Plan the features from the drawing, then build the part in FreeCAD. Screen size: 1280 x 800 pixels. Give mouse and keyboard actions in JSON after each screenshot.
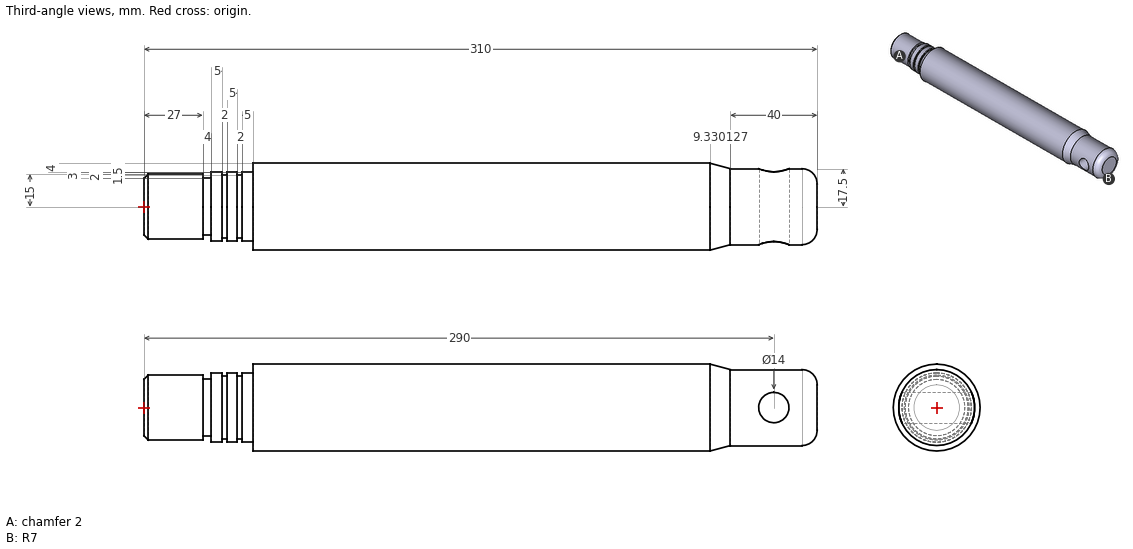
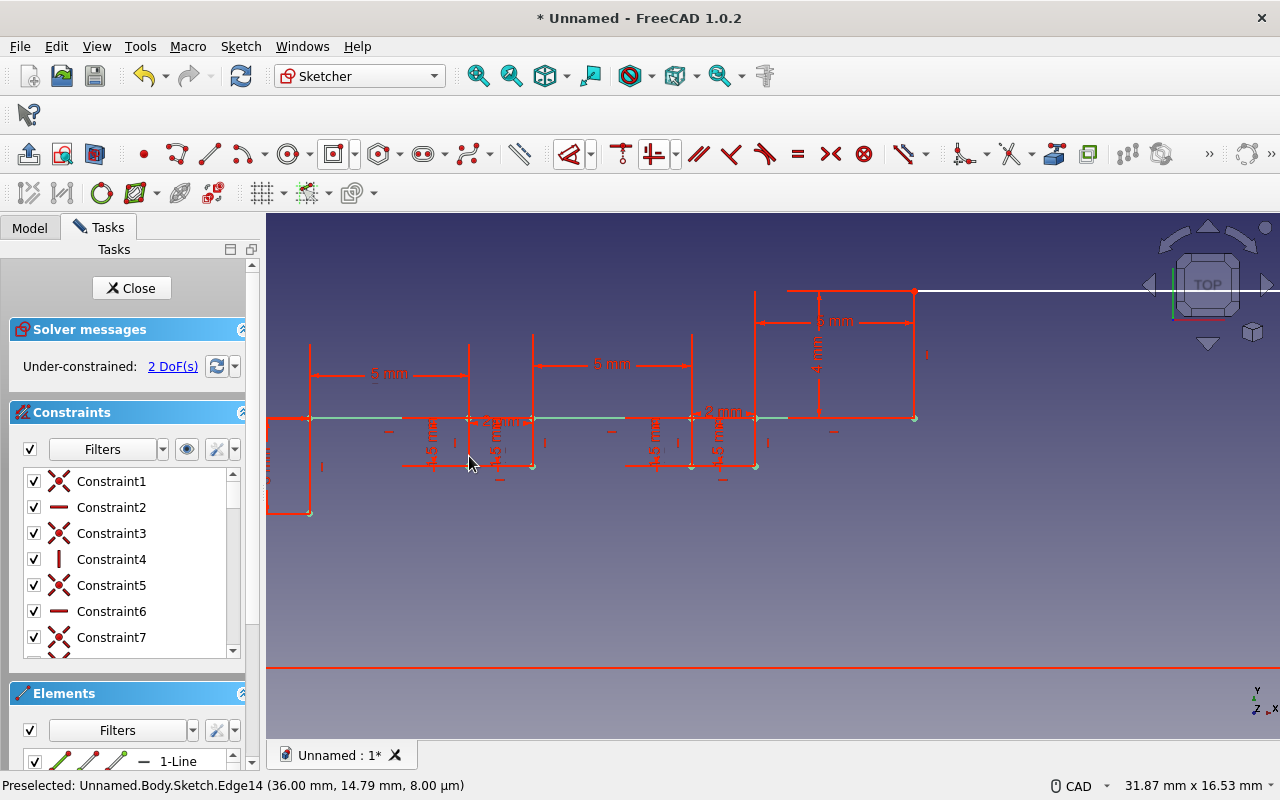
{"action": "scroll", "coordinate": [475, 467], "scroll_direction": "down", "scroll_amount": 14}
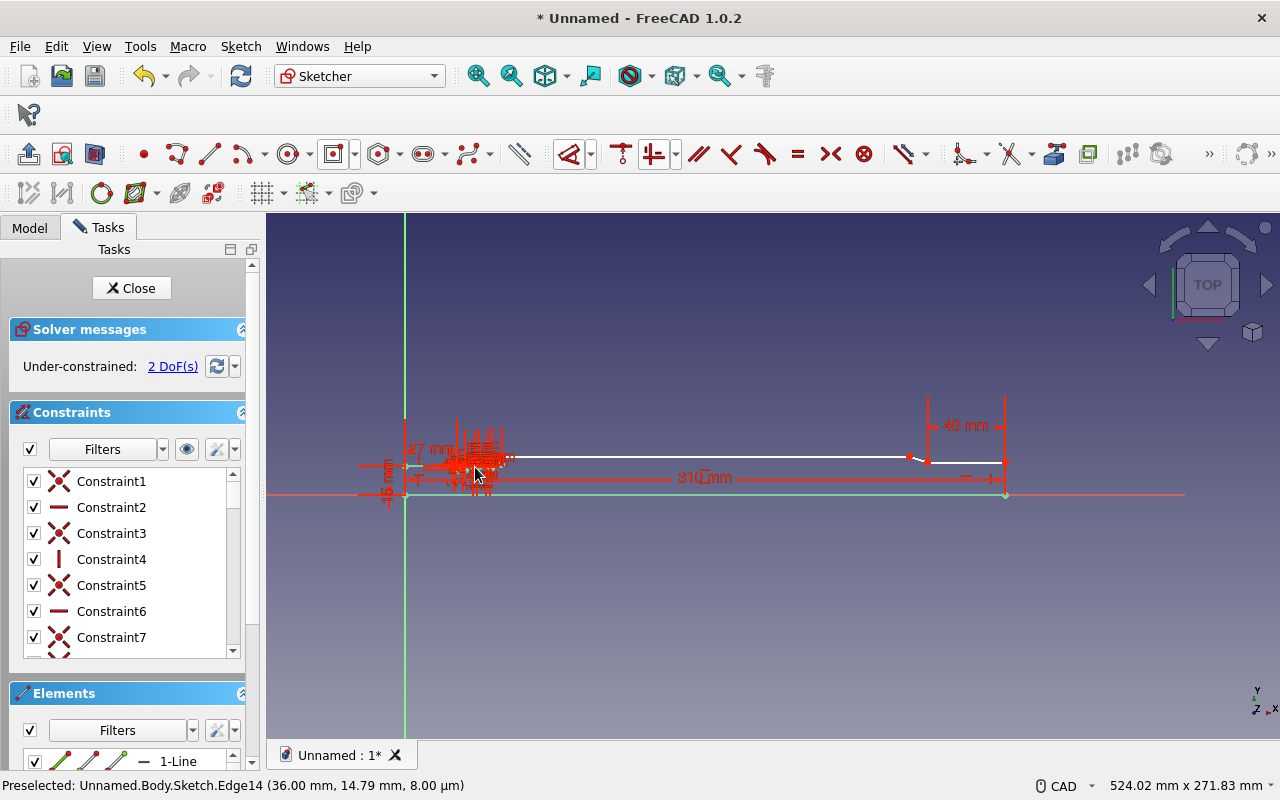
{"action": "scroll", "coordinate": [1005, 486], "scroll_direction": "up", "scroll_amount": 2}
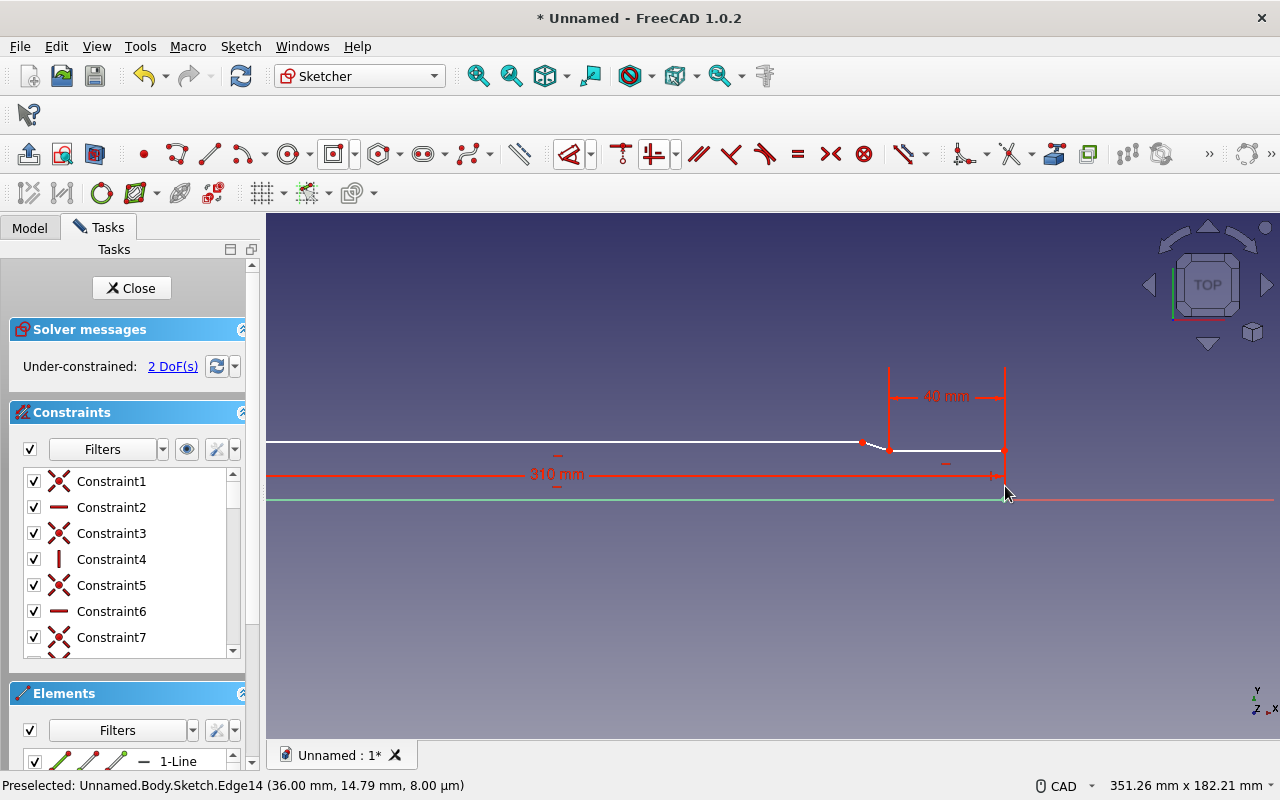
{"action": "left_click", "coordinate": [1005, 485]}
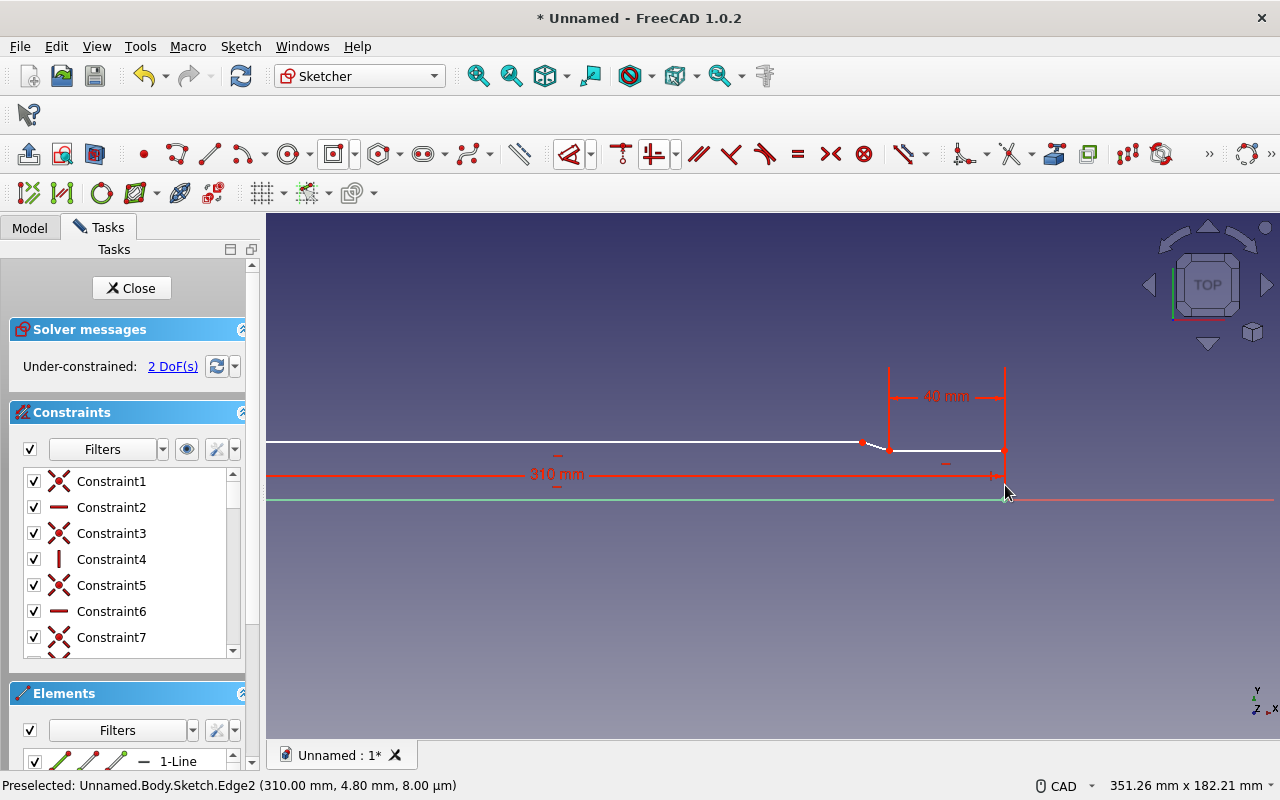
{"action": "key", "text": "i"}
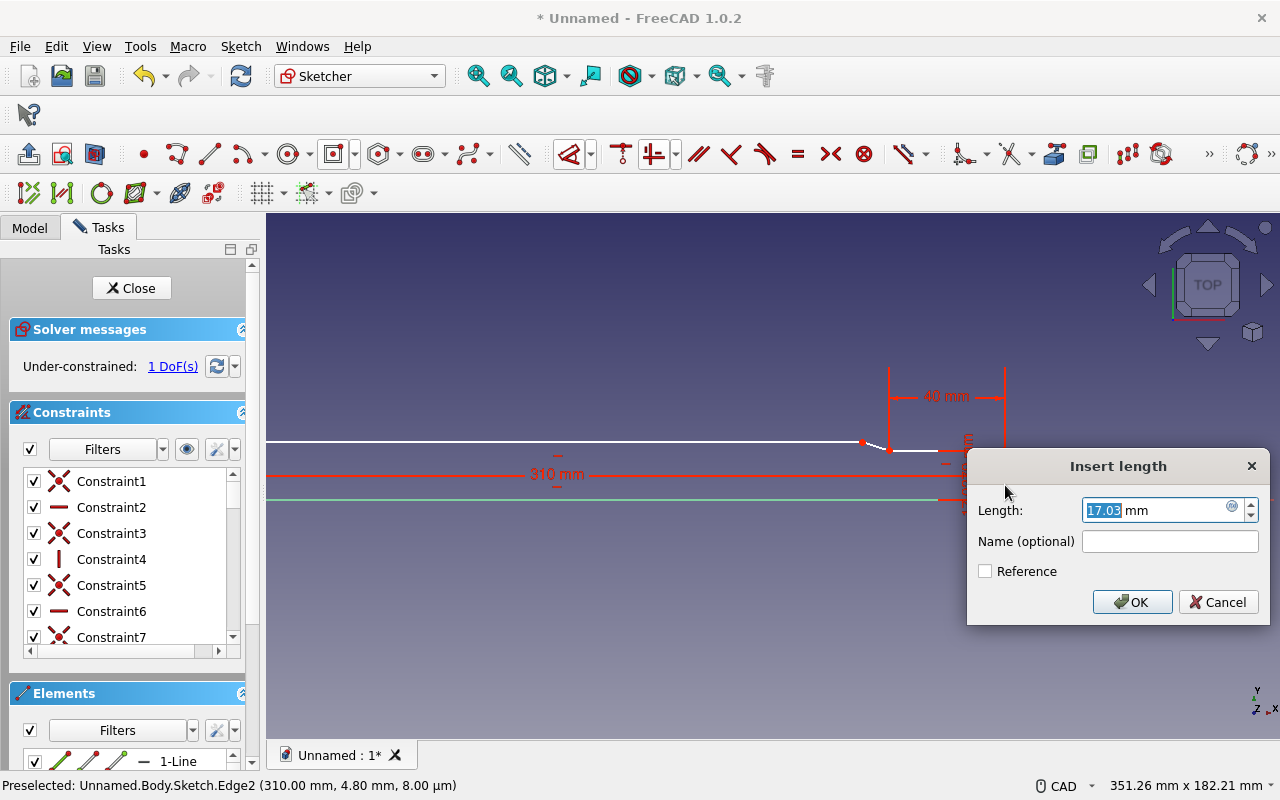
{"action": "type", "text": "17.5"}
{"action": "key", "text": "Return"}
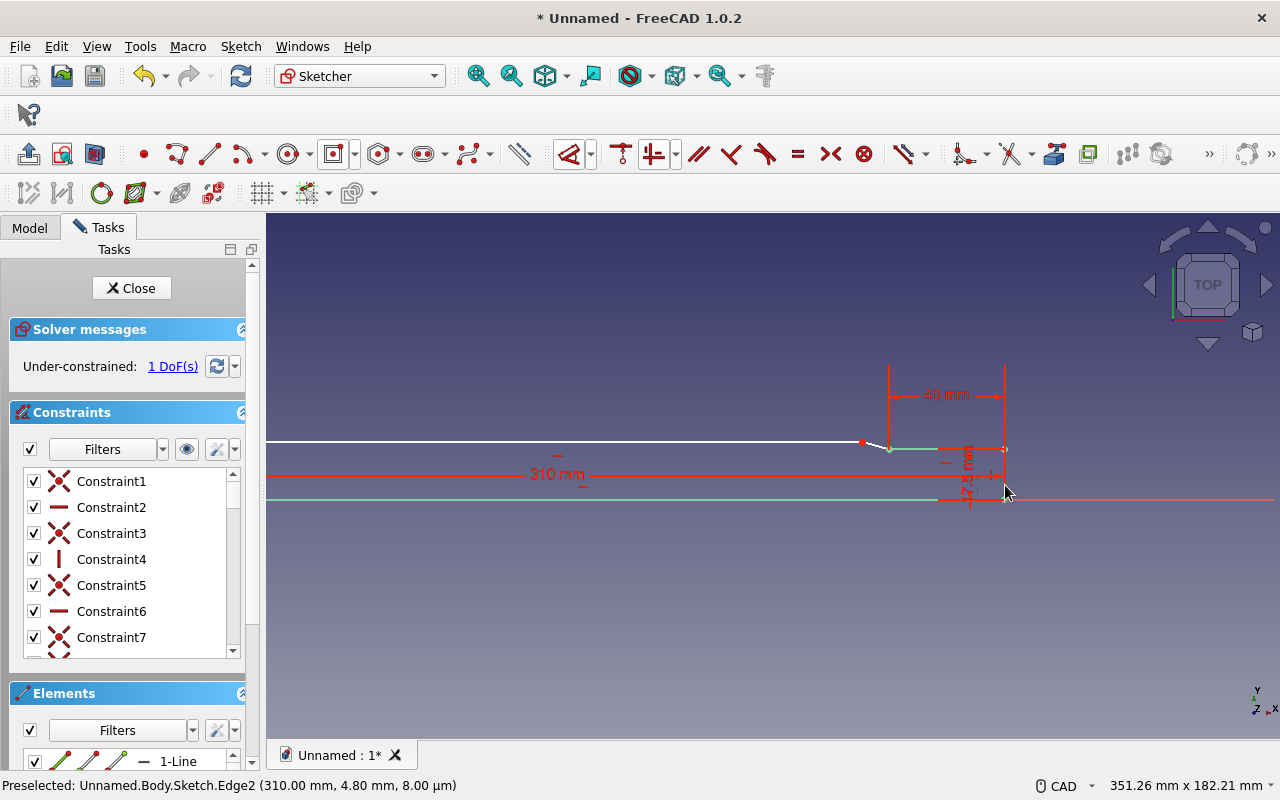
{"action": "scroll", "coordinate": [879, 446], "scroll_direction": "up", "scroll_amount": 2}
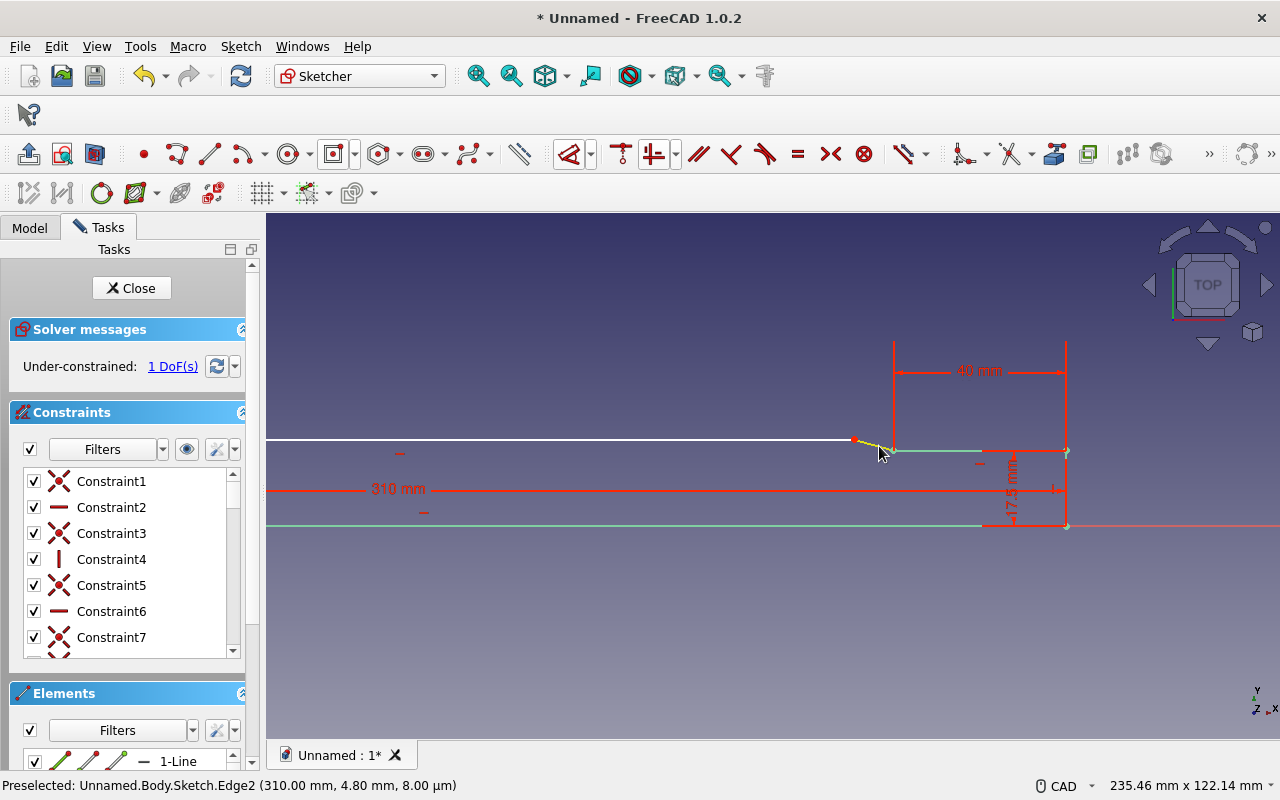
{"action": "left_click", "coordinate": [878, 446]}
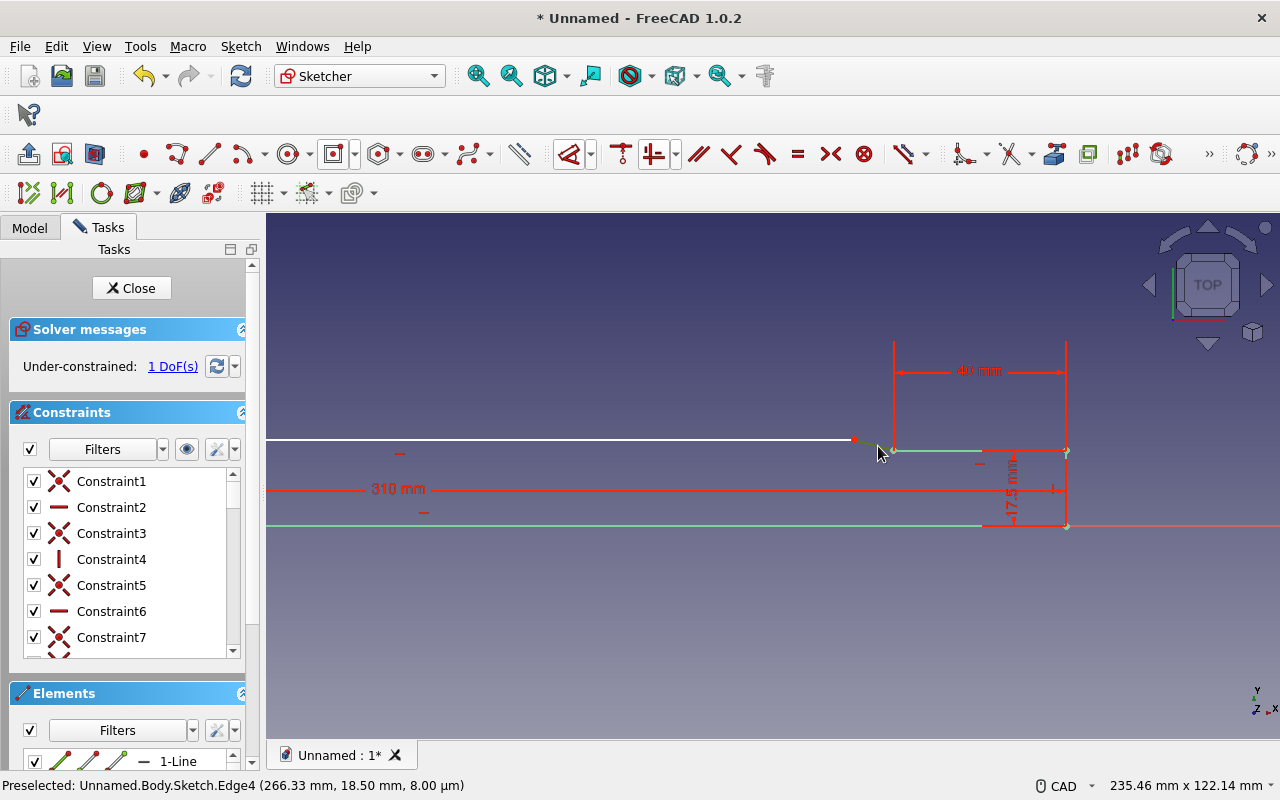
{"action": "left_click", "coordinate": [590, 154]}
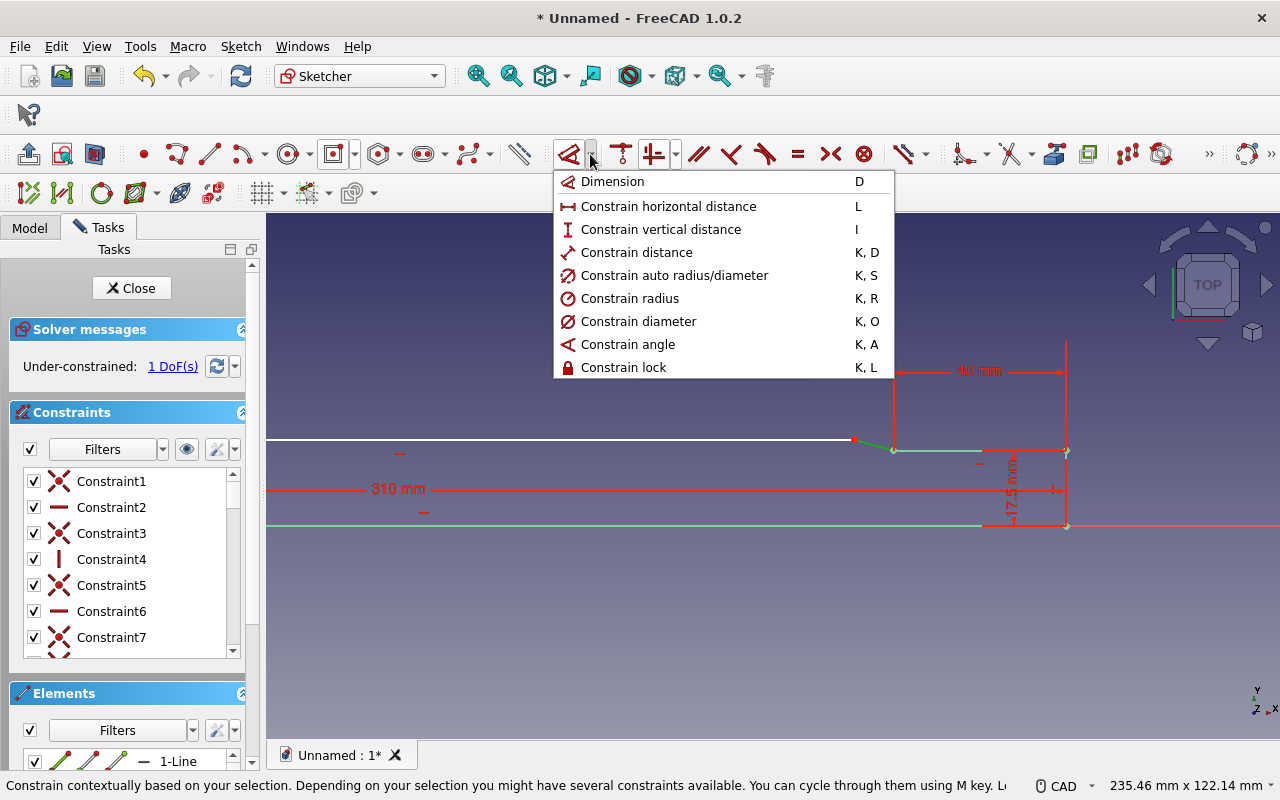
{"action": "left_click", "coordinate": [724, 206]}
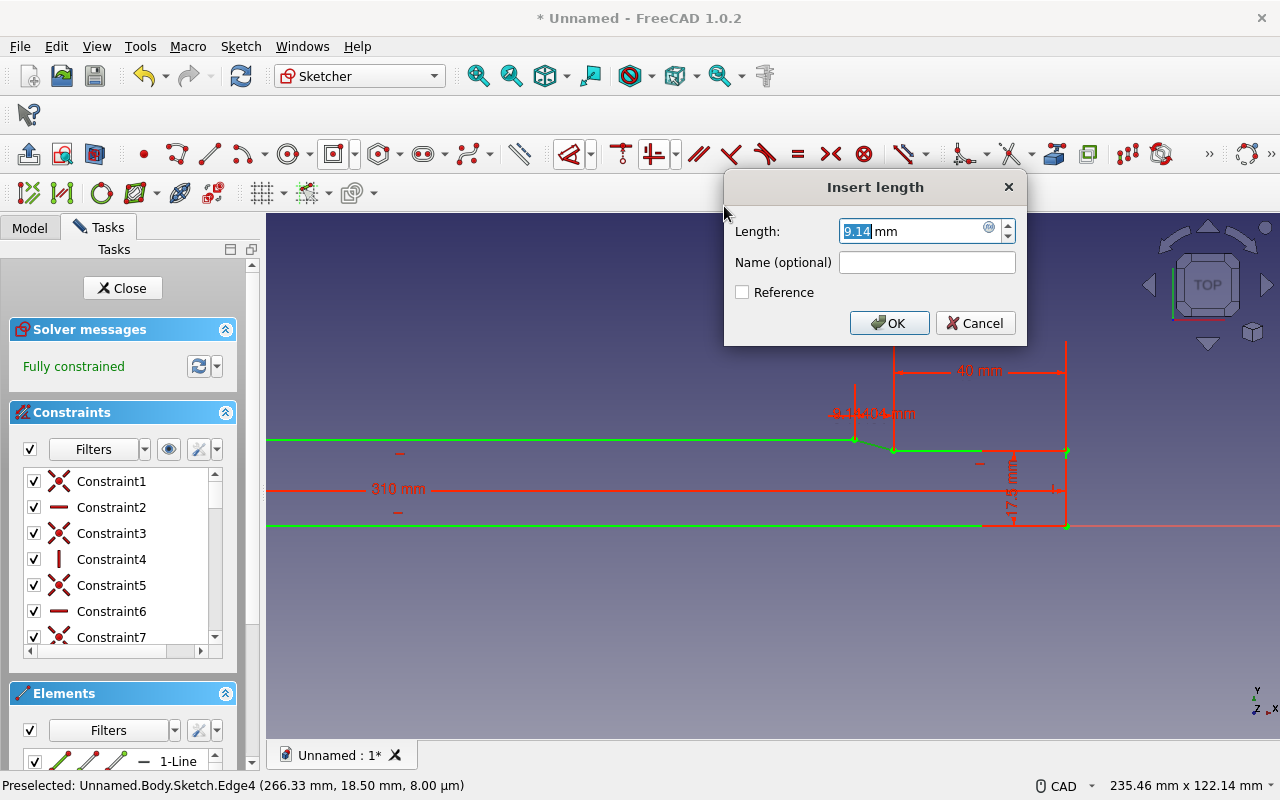
{"action": "type", "text": "9.330127"}
{"action": "key", "text": "Return"}